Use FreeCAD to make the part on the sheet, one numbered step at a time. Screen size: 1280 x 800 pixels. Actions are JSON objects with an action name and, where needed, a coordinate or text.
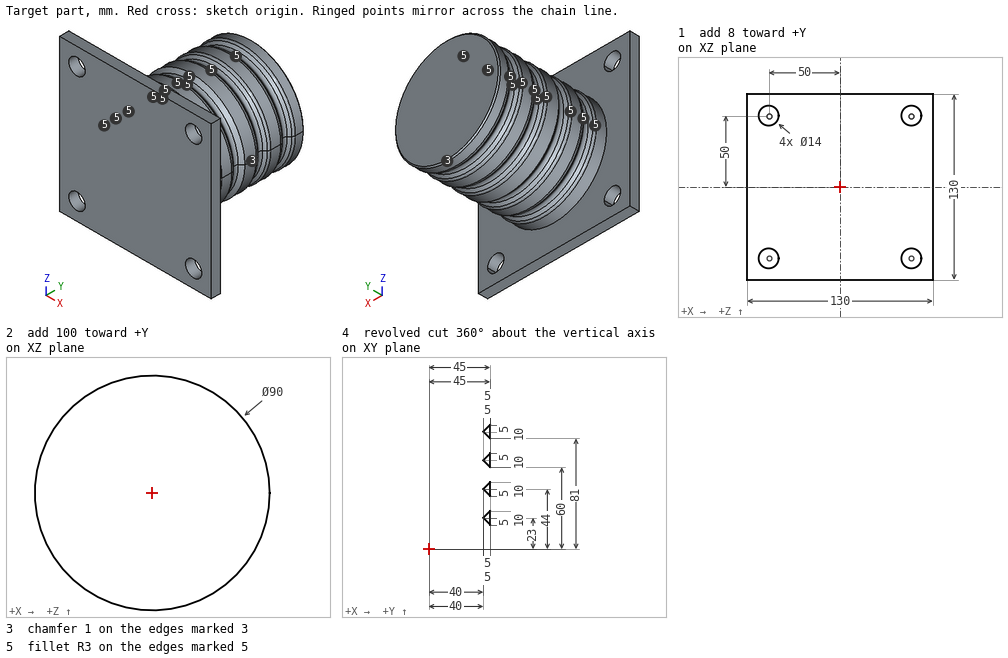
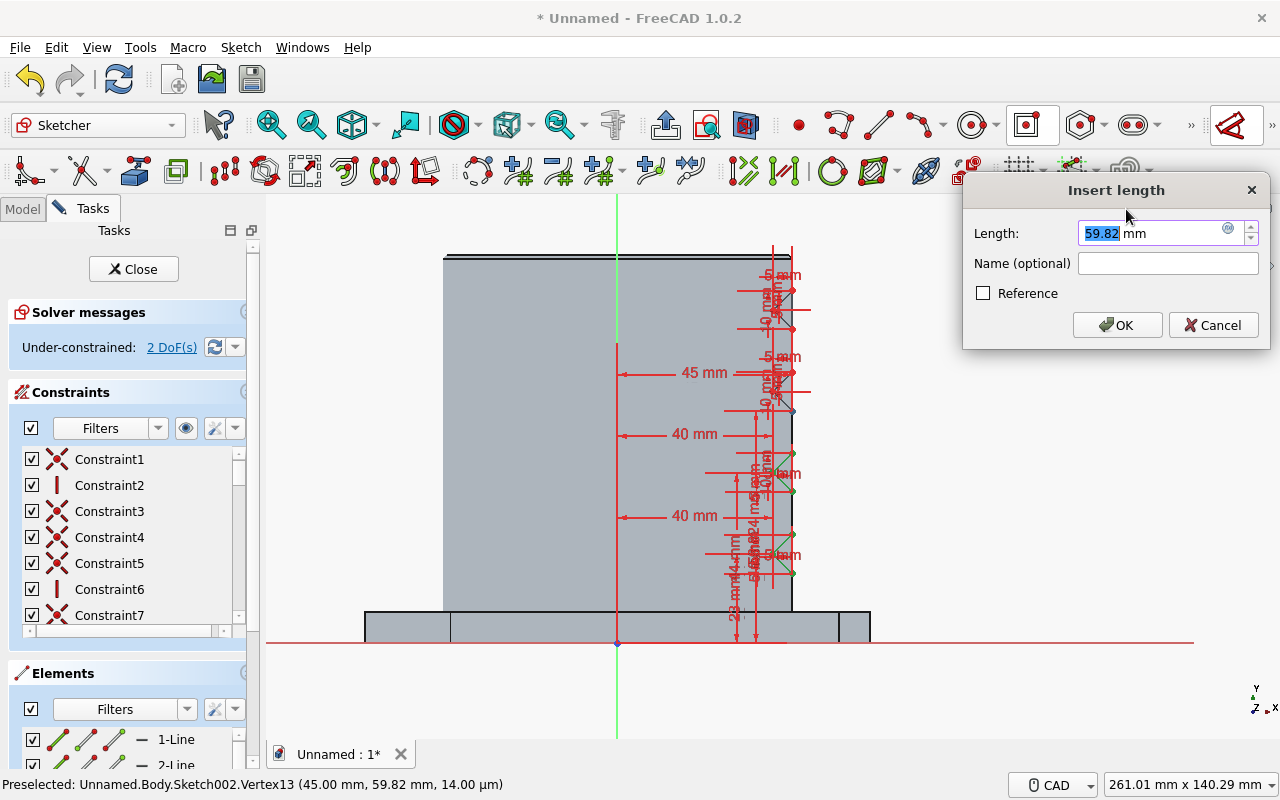
{"action": "type", "text": "60"}
{"action": "key", "text": "Return"}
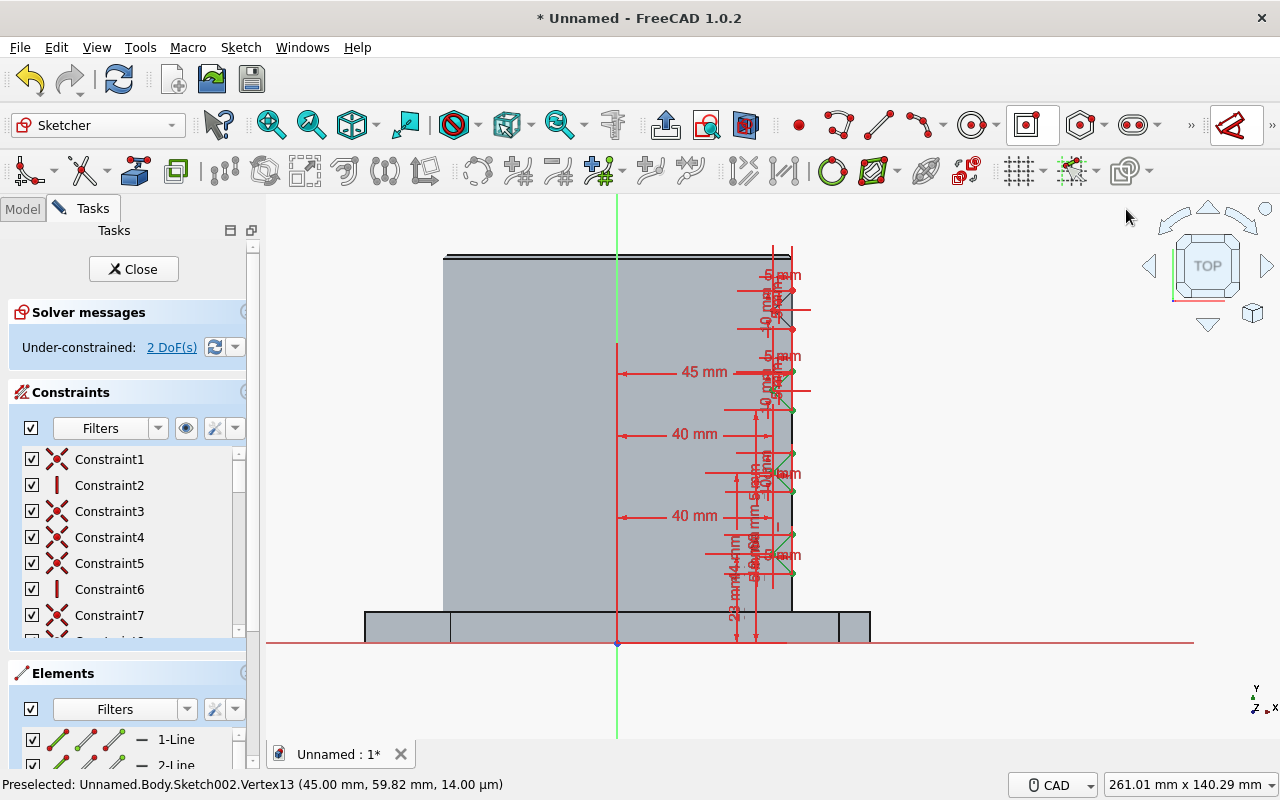
{"action": "left_click", "coordinate": [792, 329]}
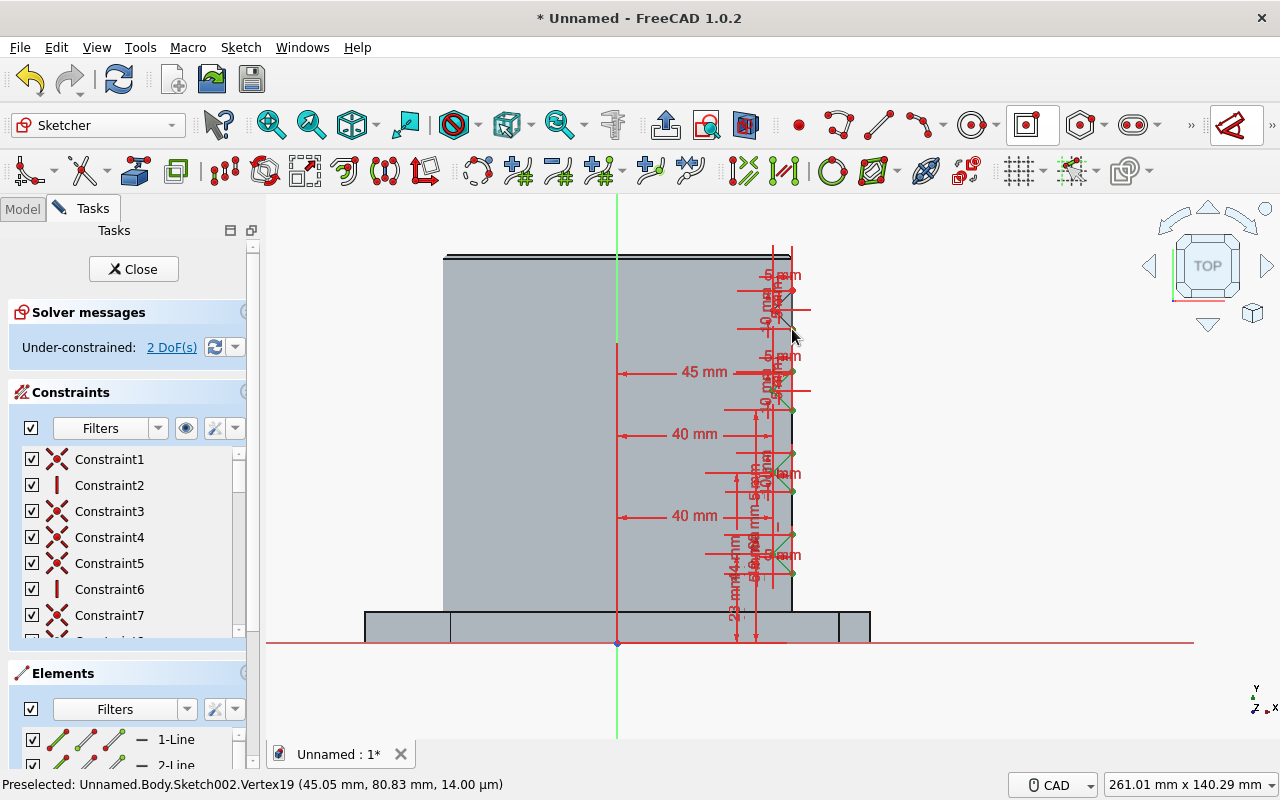
{"action": "key", "text": "l"}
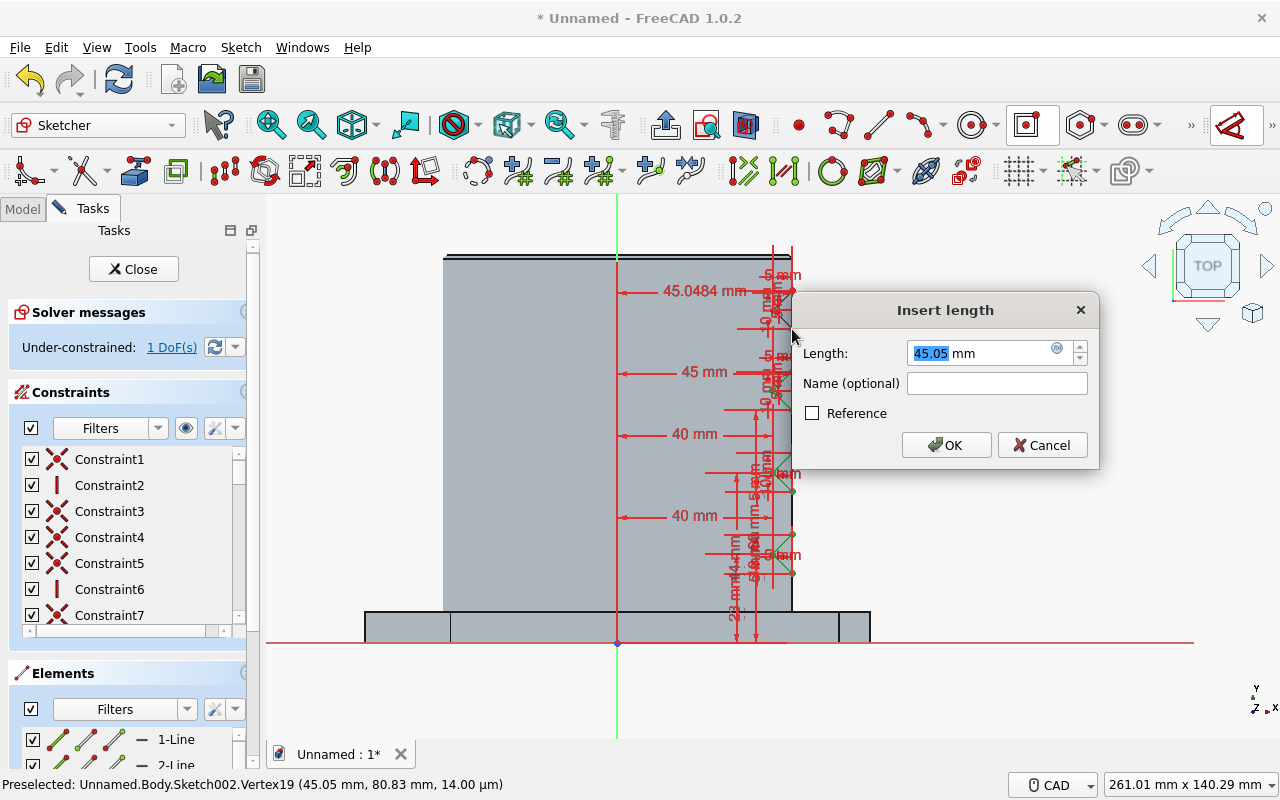
{"action": "type", "text": "45"}
{"action": "key", "text": "Return"}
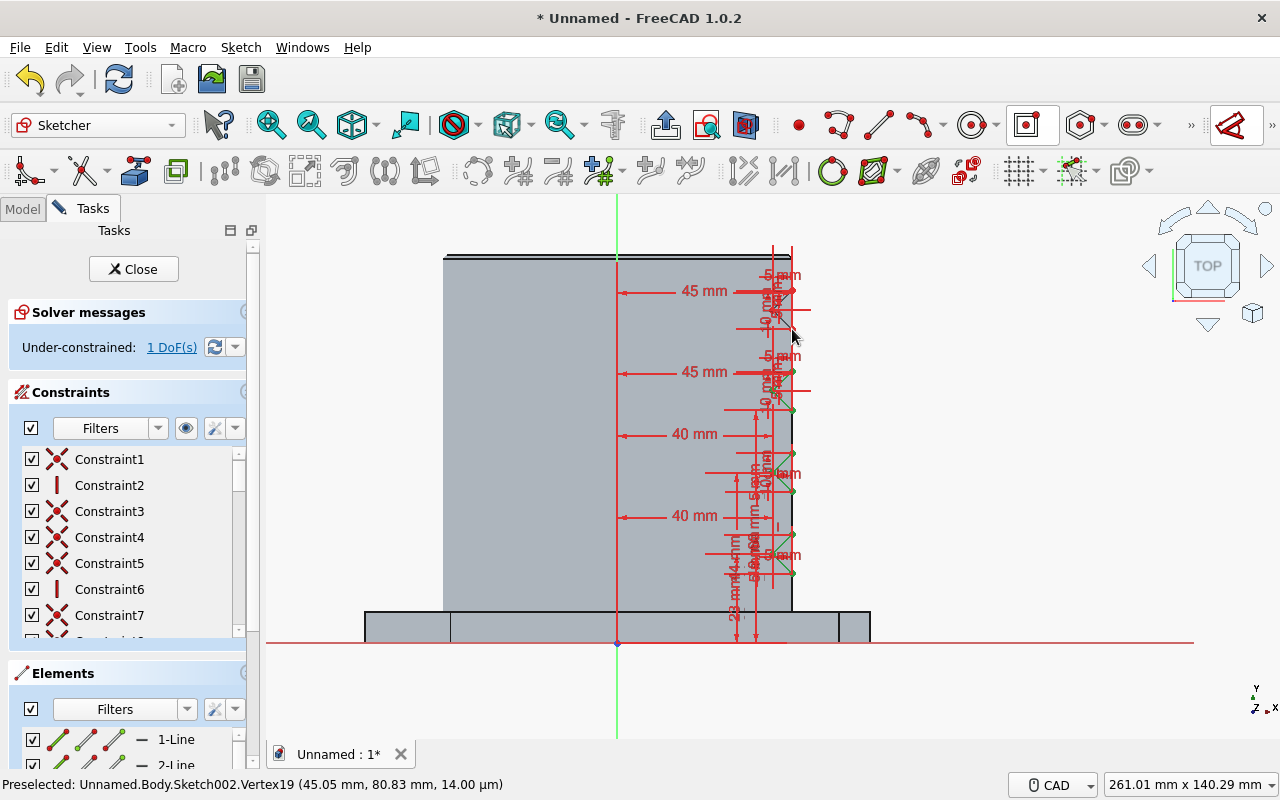
{"action": "left_click", "coordinate": [792, 329]}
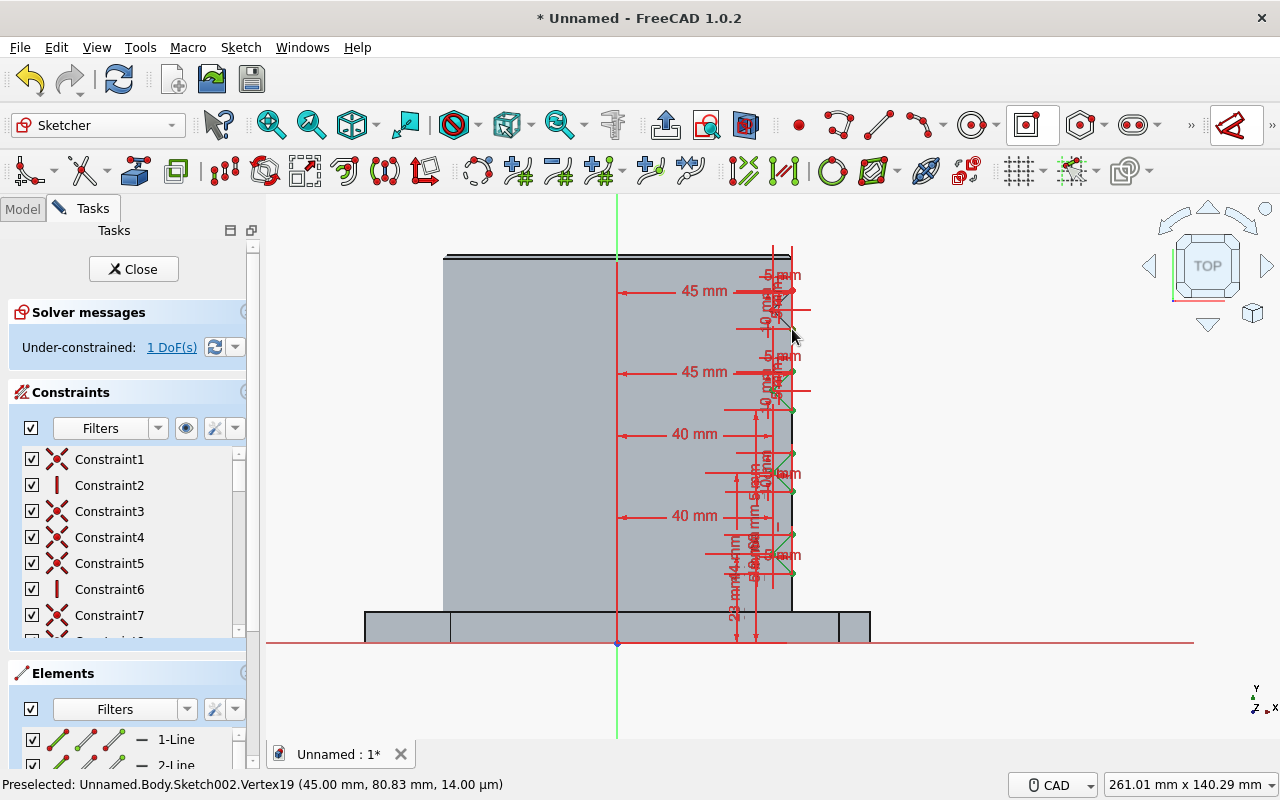
{"action": "key", "text": "i"}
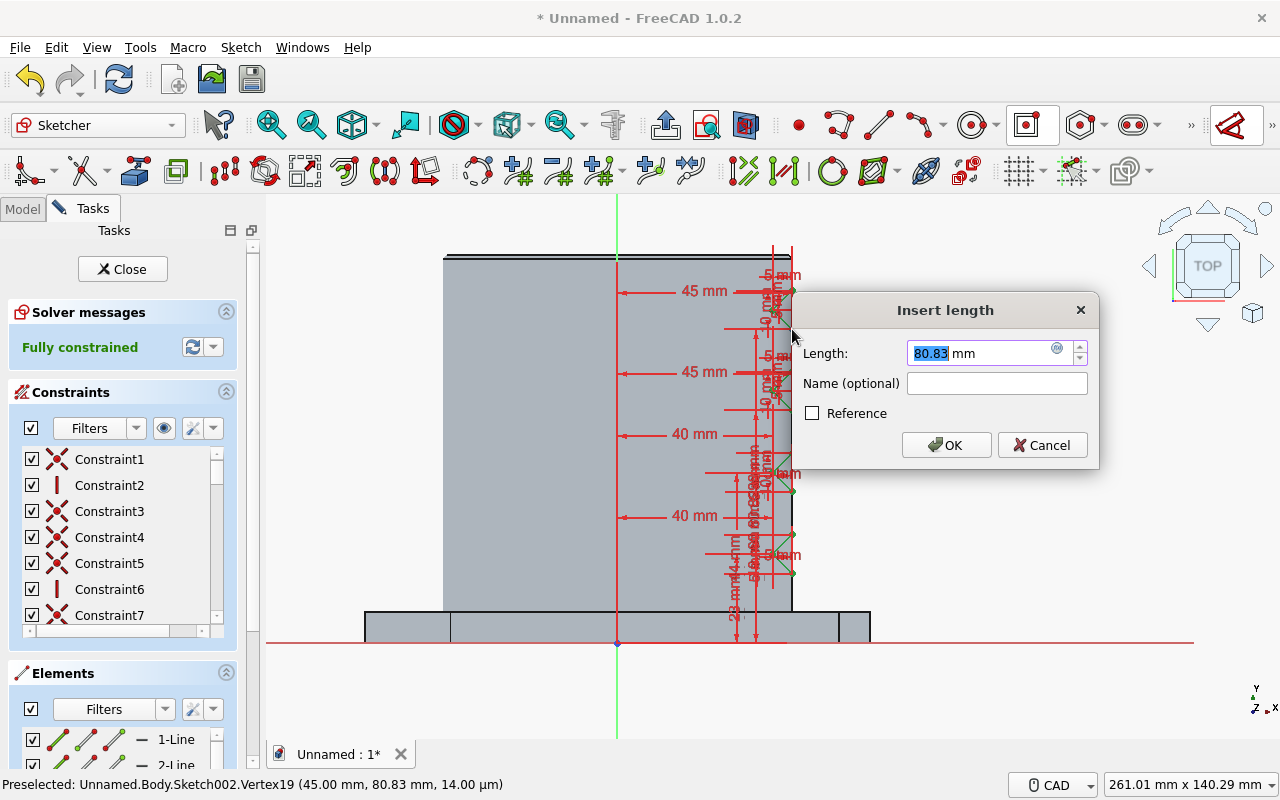
{"action": "type", "text": "81"}
{"action": "key", "text": "Return"}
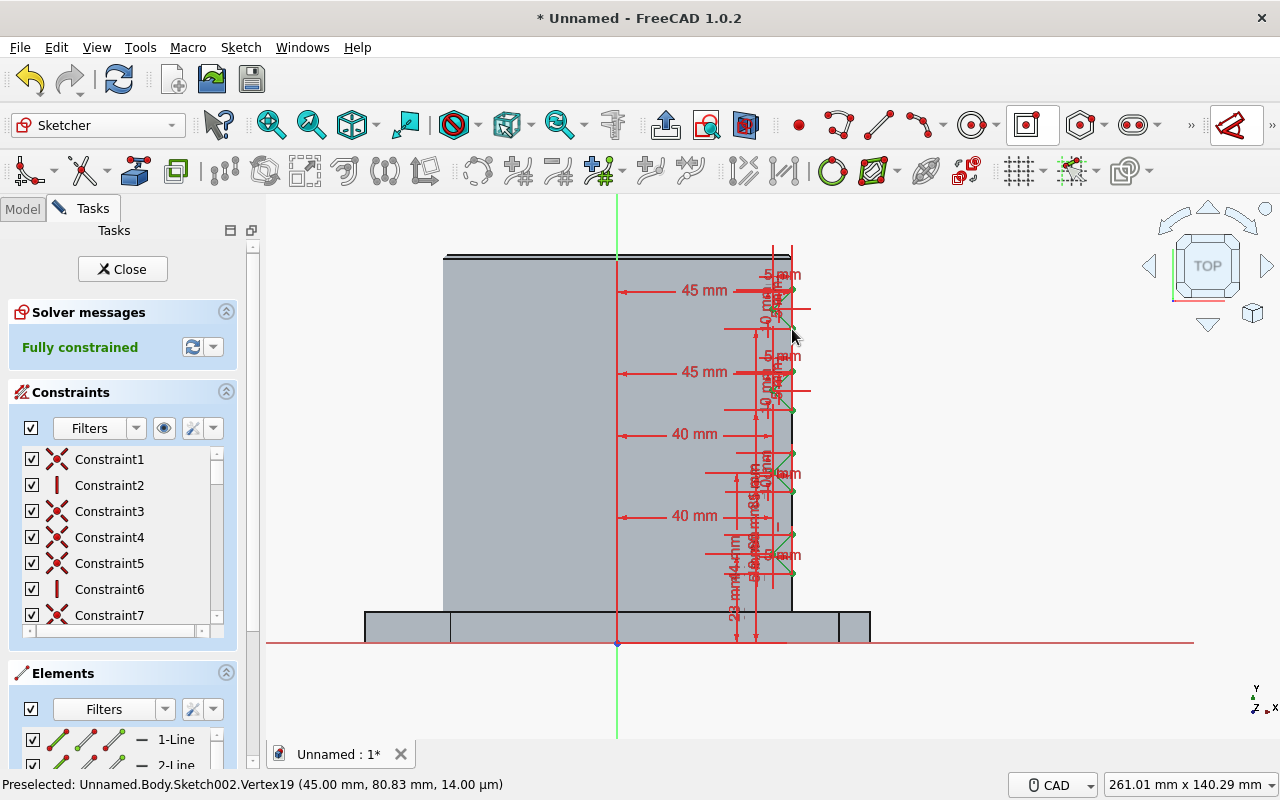
{"action": "left_click", "coordinate": [123, 269]}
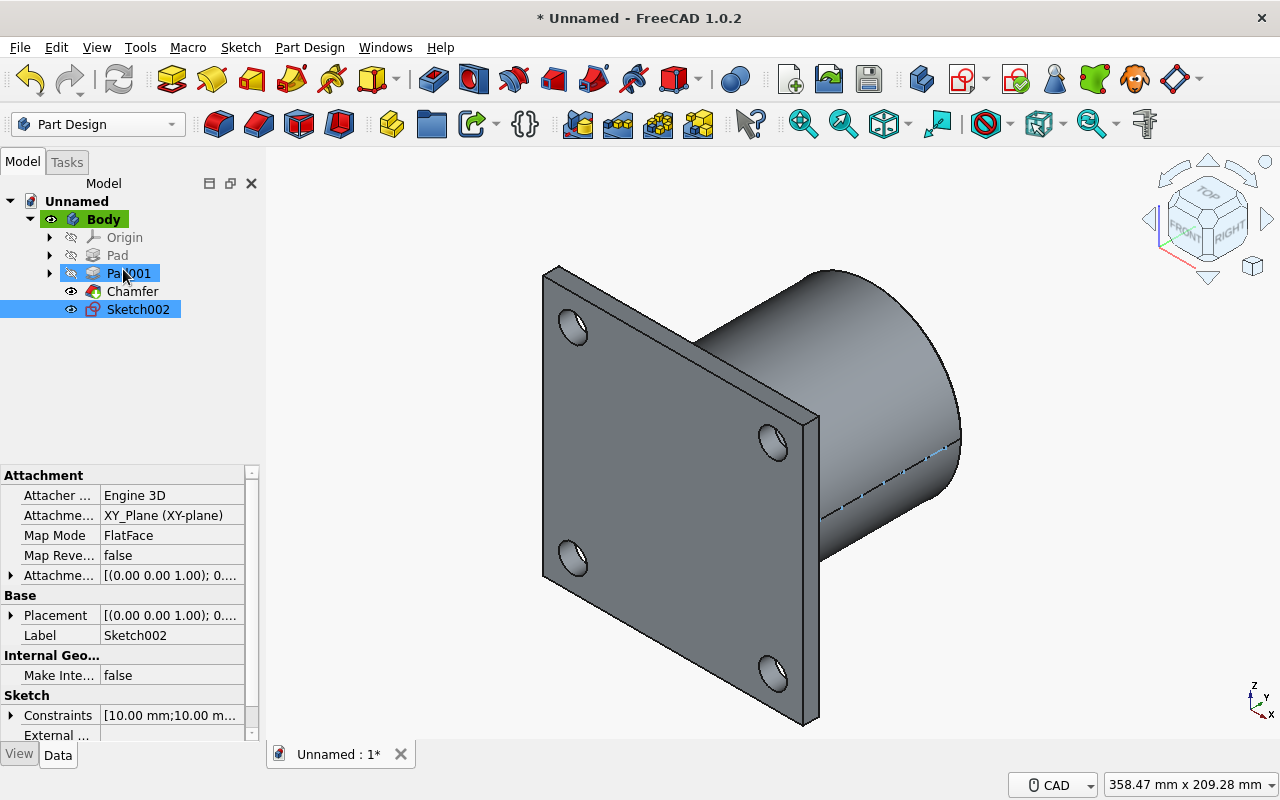
{"action": "left_click", "coordinate": [514, 80]}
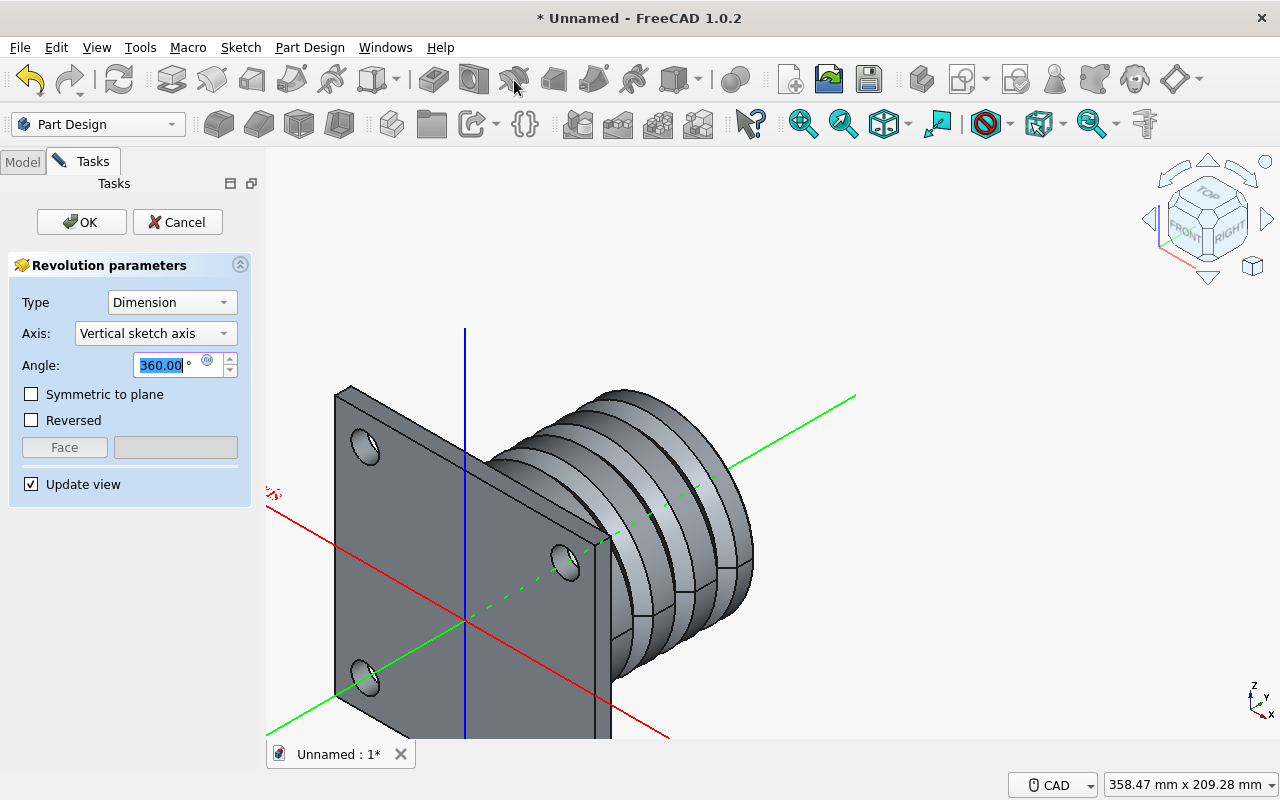
{"action": "left_click", "coordinate": [82, 222]}